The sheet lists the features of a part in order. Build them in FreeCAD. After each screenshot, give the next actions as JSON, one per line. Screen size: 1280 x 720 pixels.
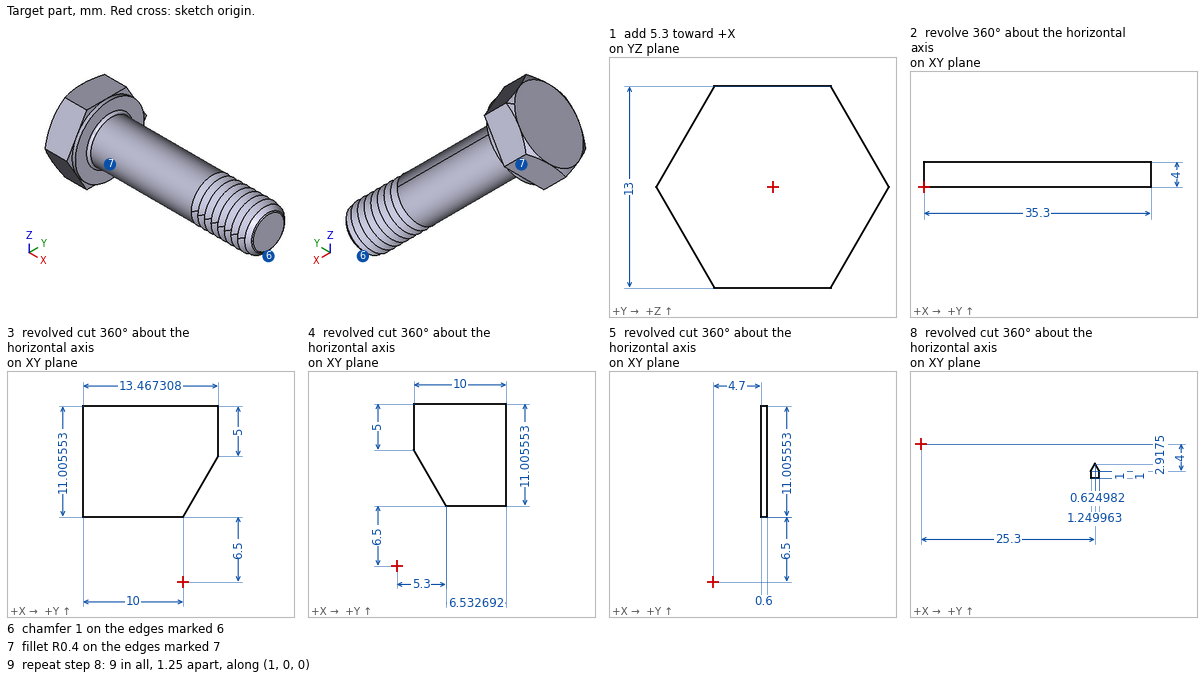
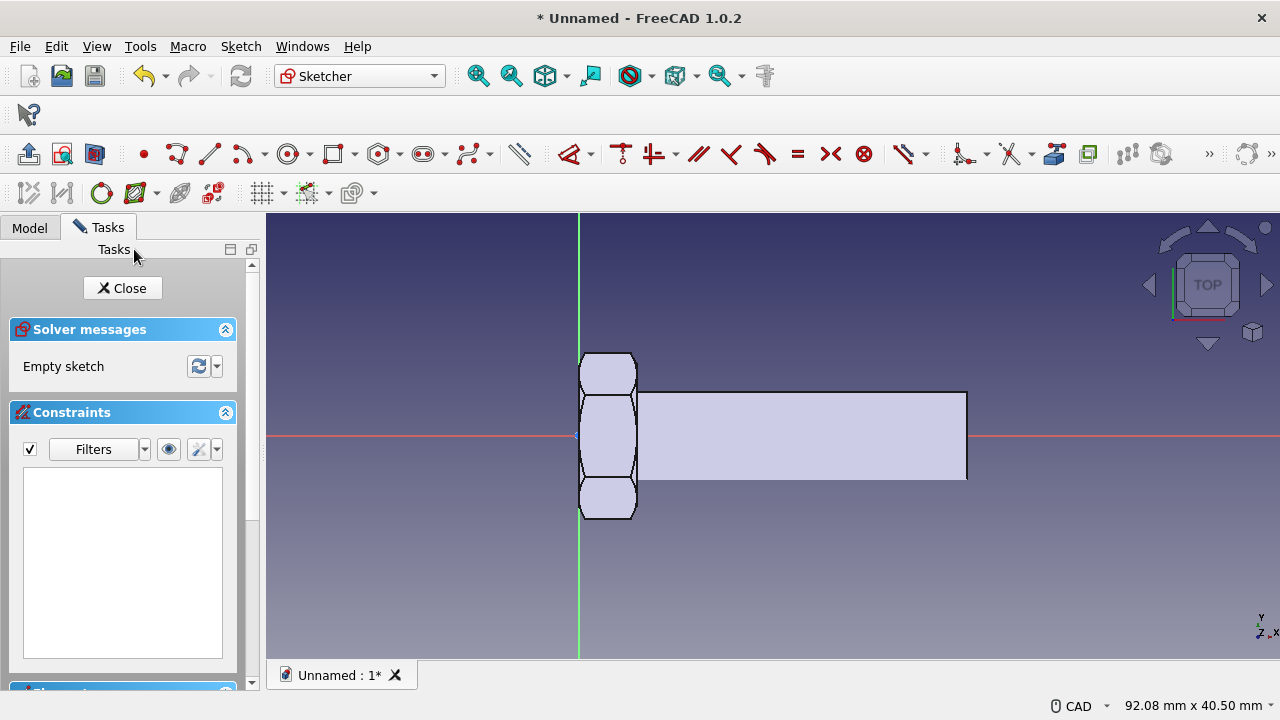
{"action": "left_click", "coordinate": [95, 154]}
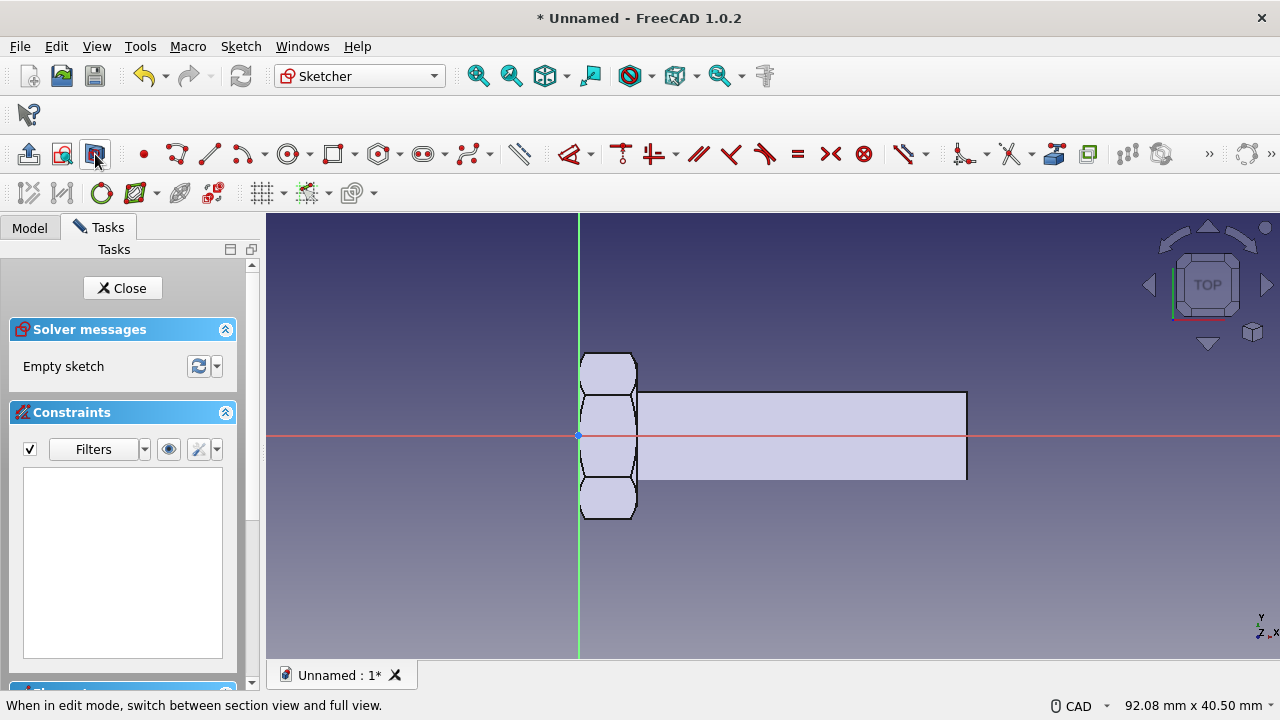
{"action": "scroll", "coordinate": [1115, 631], "scroll_direction": "down", "scroll_amount": 1}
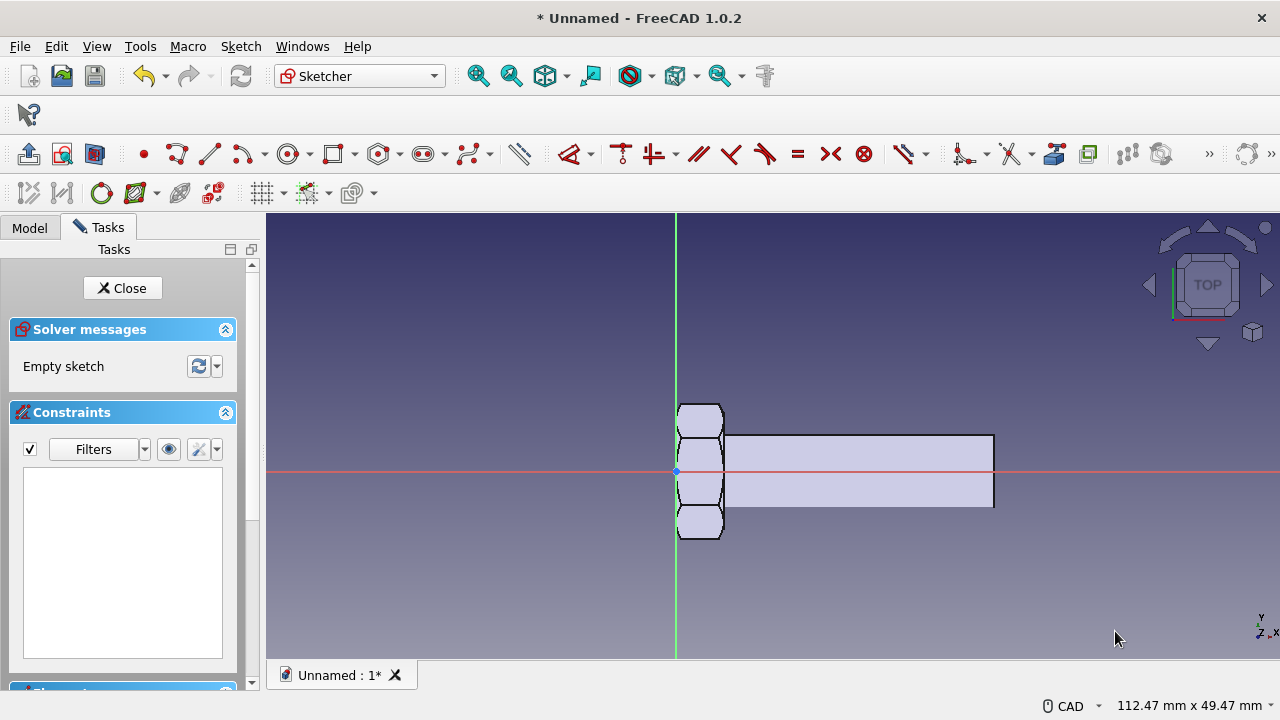
{"action": "scroll", "coordinate": [694, 340], "scroll_direction": "up", "scroll_amount": 3}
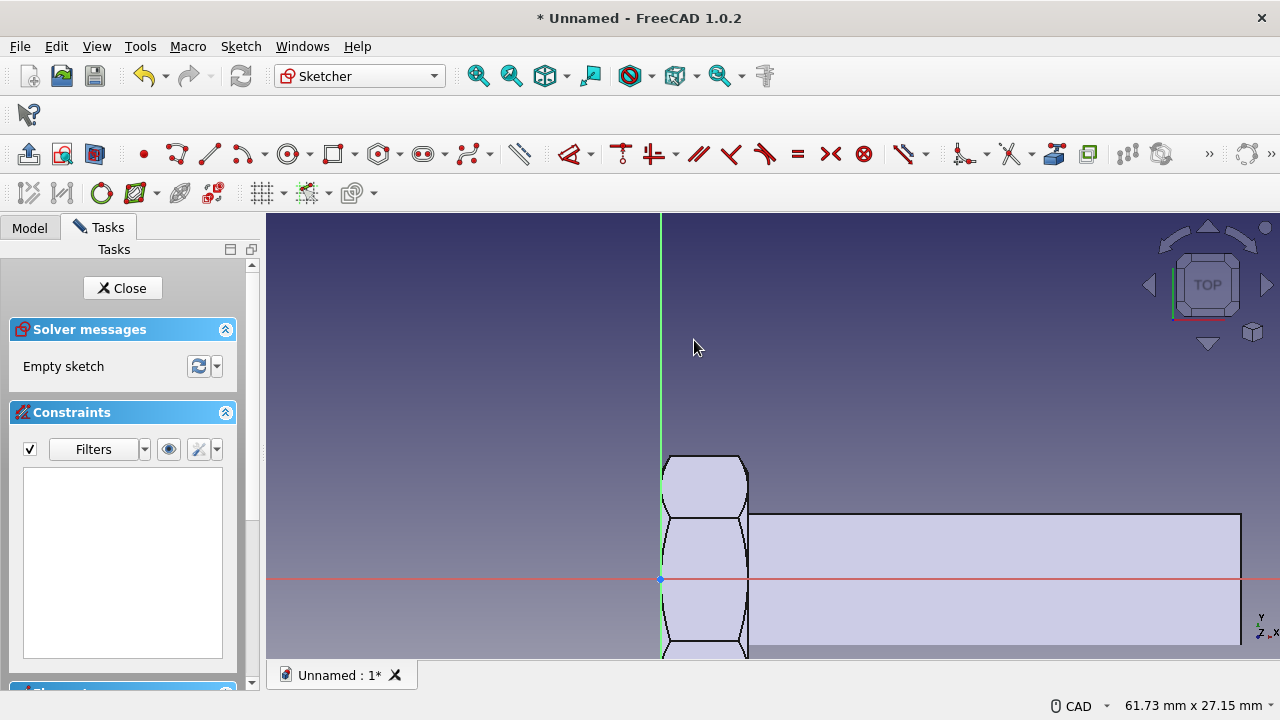
{"action": "left_click", "coordinate": [332, 154]}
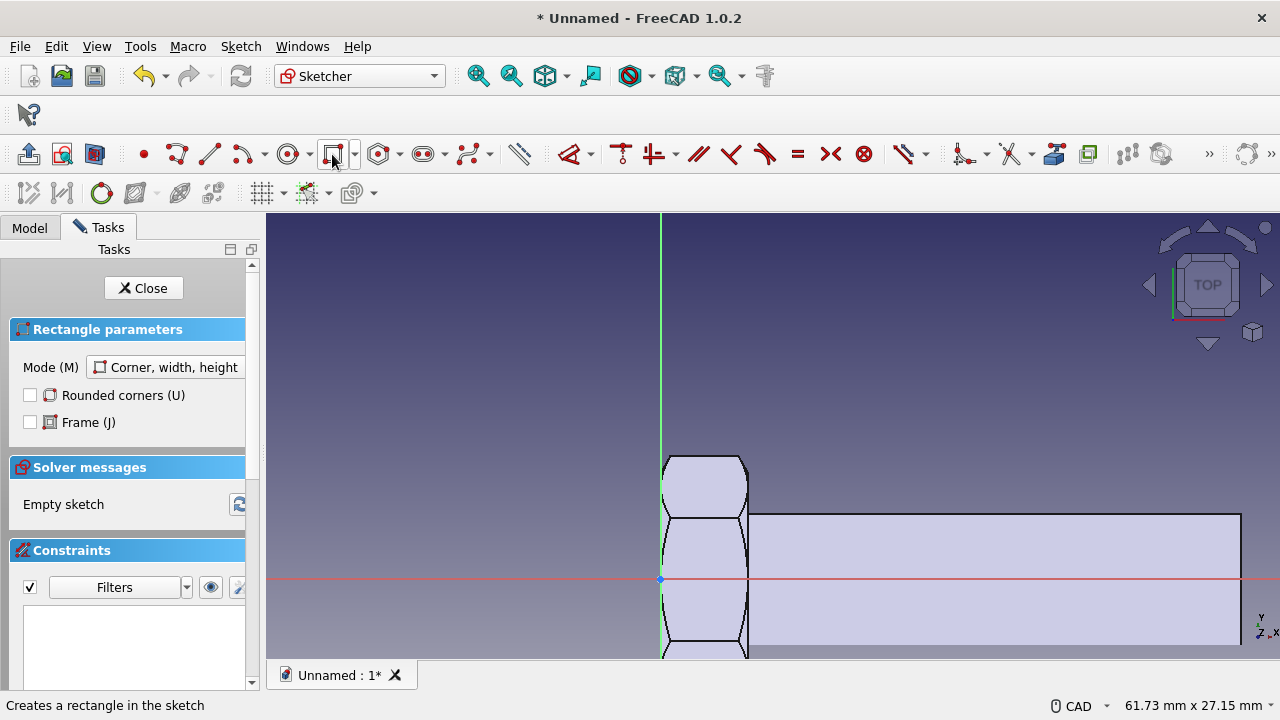
{"action": "scroll", "coordinate": [738, 292], "scroll_direction": "up", "scroll_amount": 3}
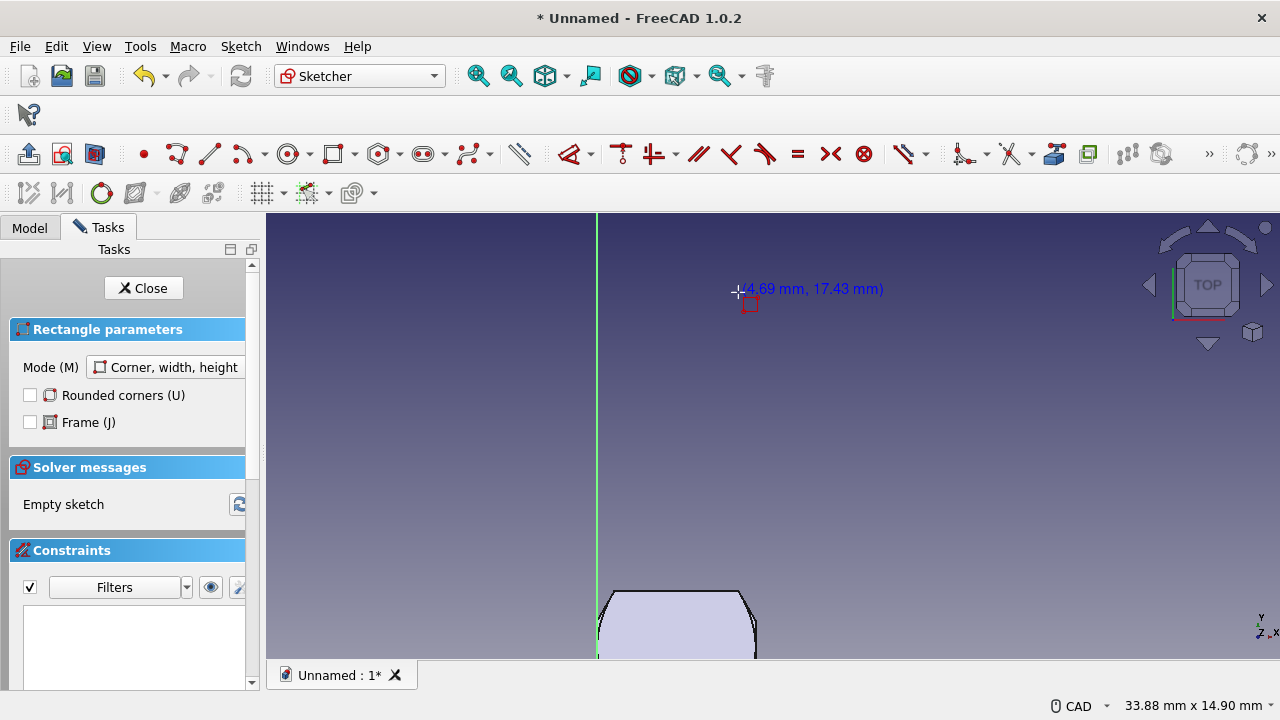
{"action": "left_click", "coordinate": [738, 292]}
{"action": "mouse_move", "coordinate": [756, 621]}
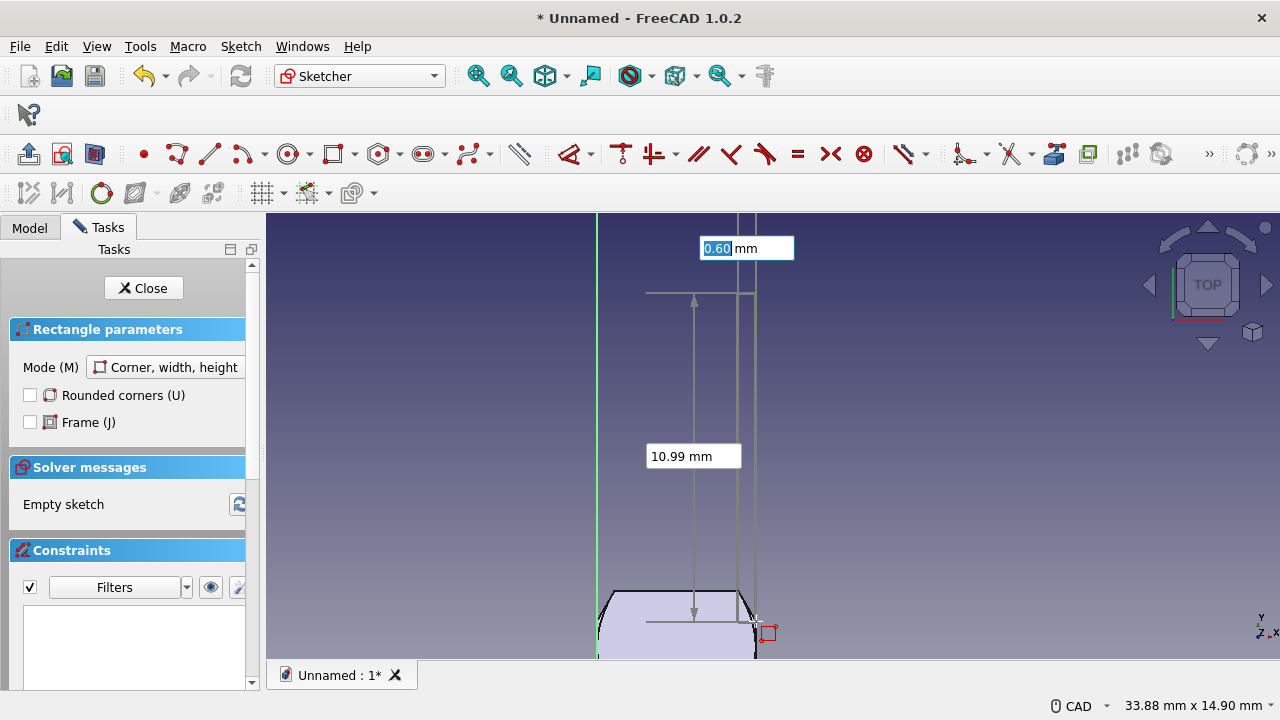
{"action": "type", "text": "0.6"}
{"action": "key", "text": "Tab"}
{"action": "type", "text": "11.005553"}
{"action": "key", "text": "Return"}
{"action": "key", "text": "Escape"}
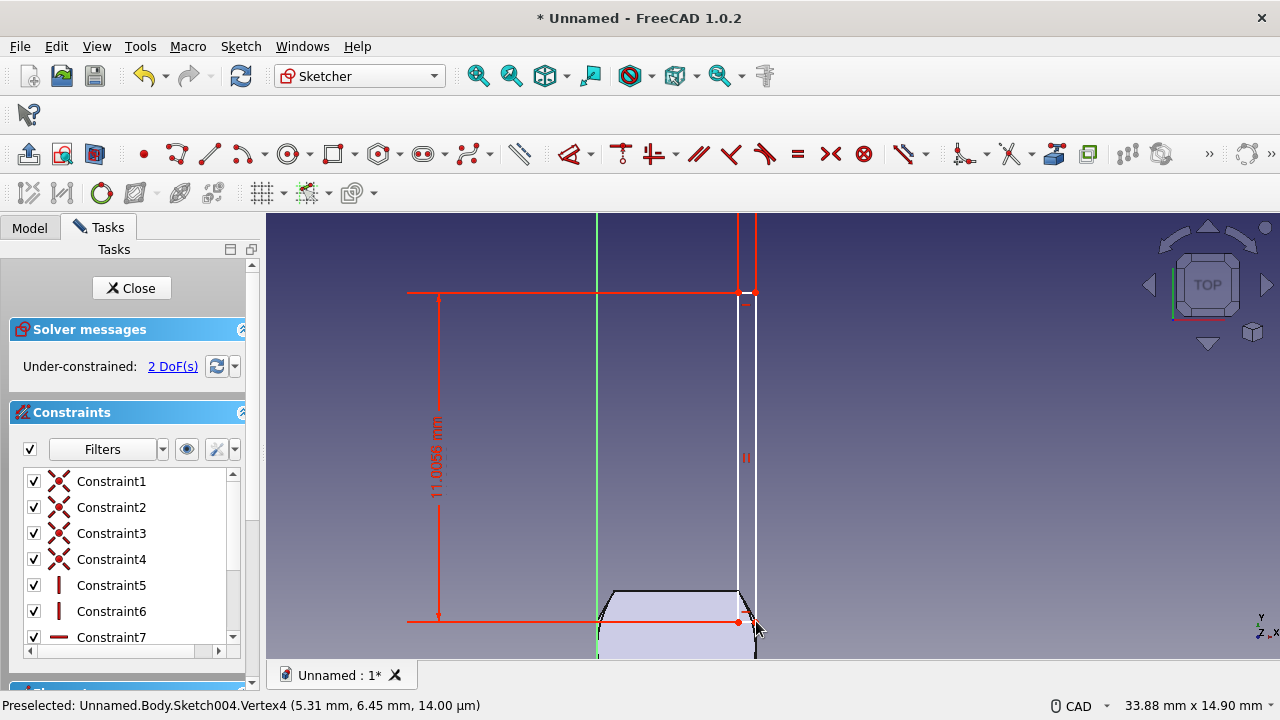
{"action": "left_click", "coordinate": [568, 154]}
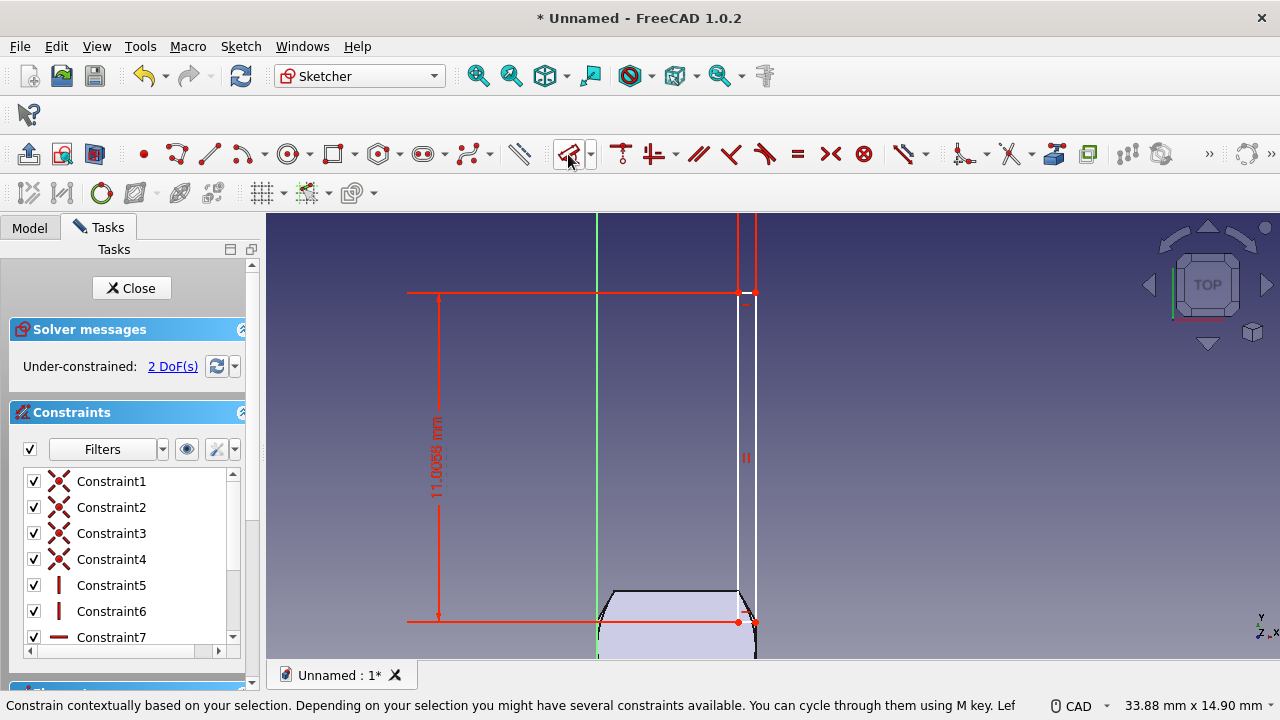
{"action": "left_click", "coordinate": [738, 293]}
{"action": "left_click", "coordinate": [668, 259]}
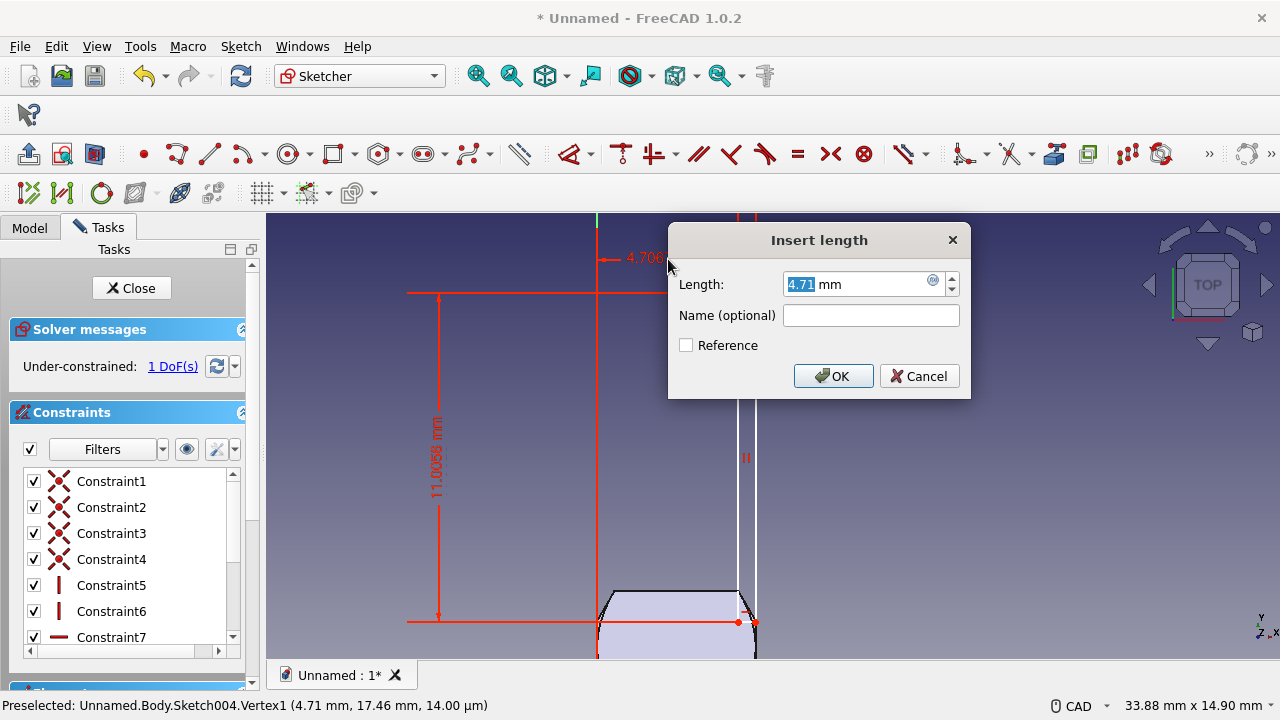
{"action": "type", "text": "4.7"}
{"action": "key", "text": "Return"}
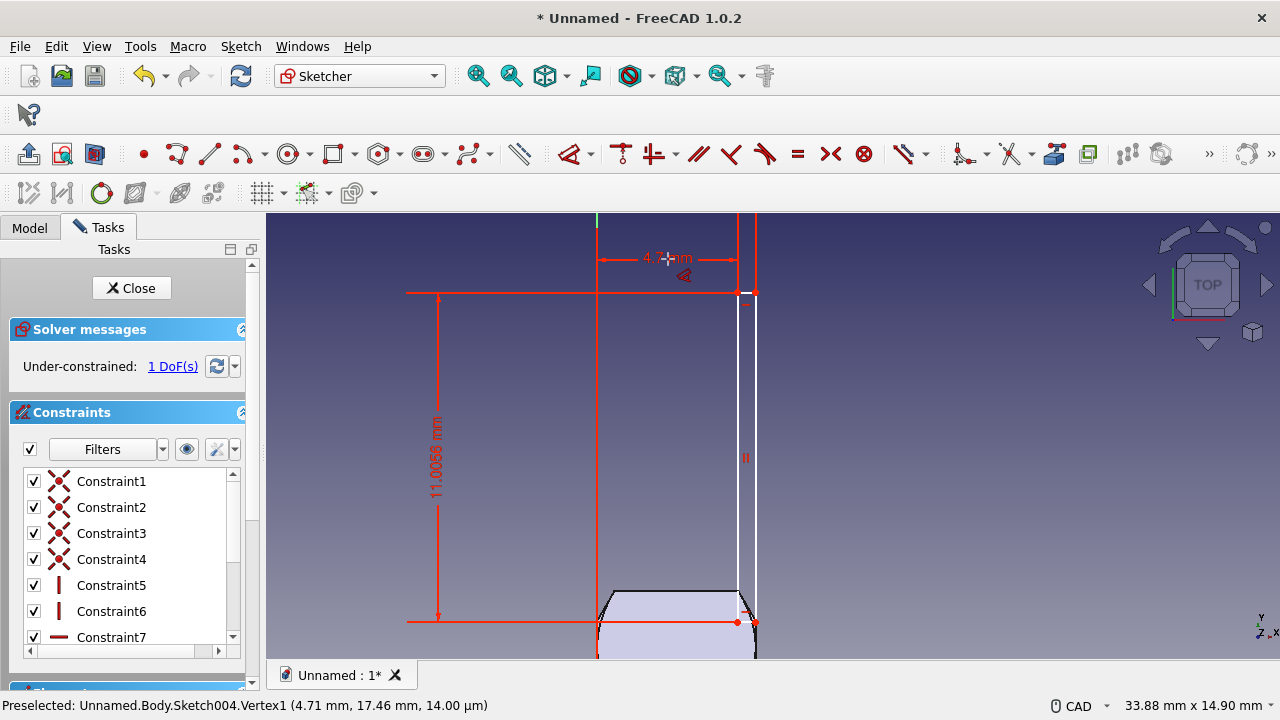
{"action": "left_click", "coordinate": [738, 622]}
{"action": "left_click", "coordinate": [563, 627]}